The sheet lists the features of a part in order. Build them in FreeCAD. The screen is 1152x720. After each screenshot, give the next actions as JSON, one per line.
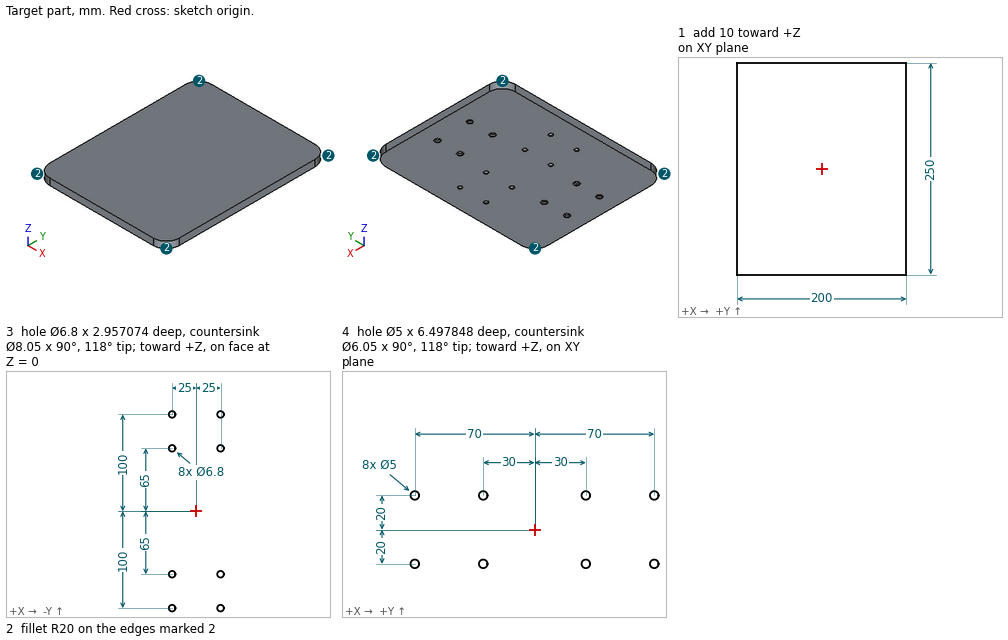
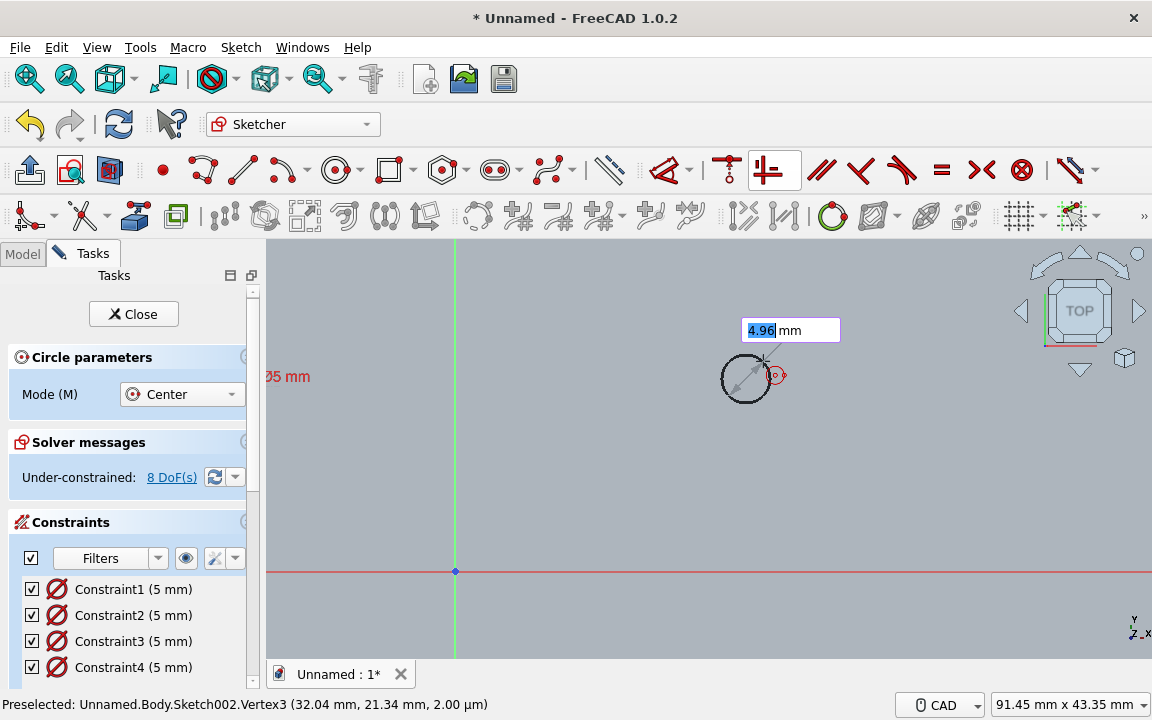
{"action": "type", "text": "5"}
{"action": "key", "text": "Return"}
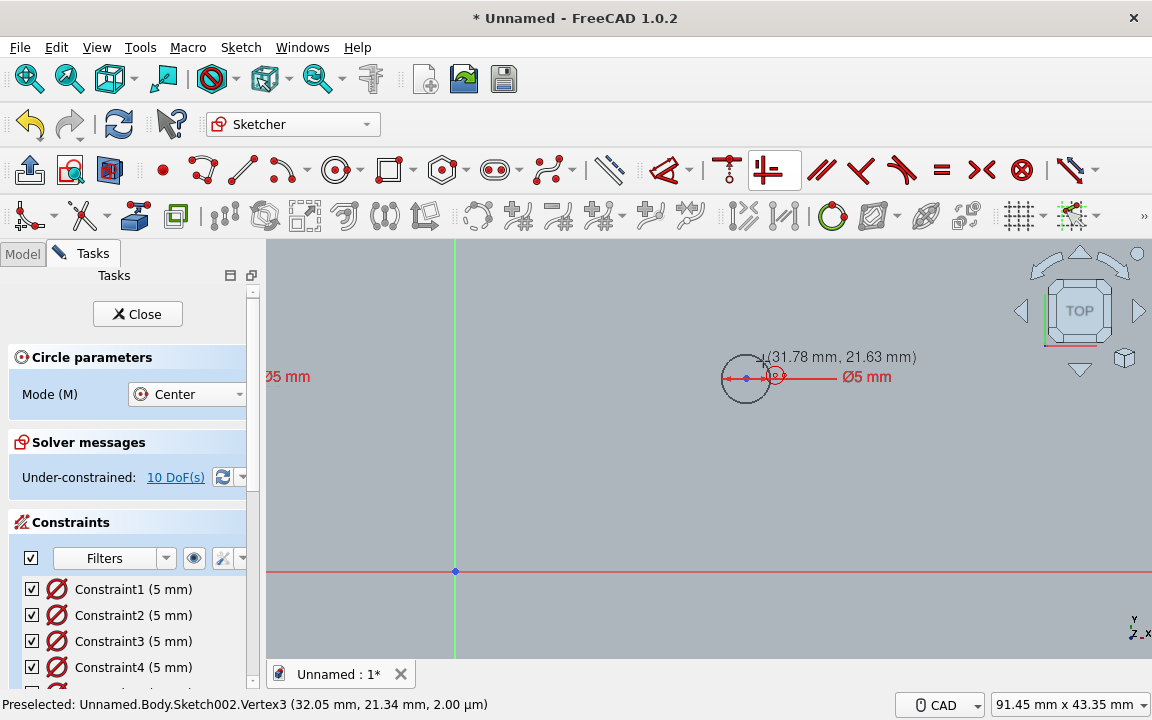
{"action": "scroll", "coordinate": [748, 378], "scroll_direction": "down", "scroll_amount": 5}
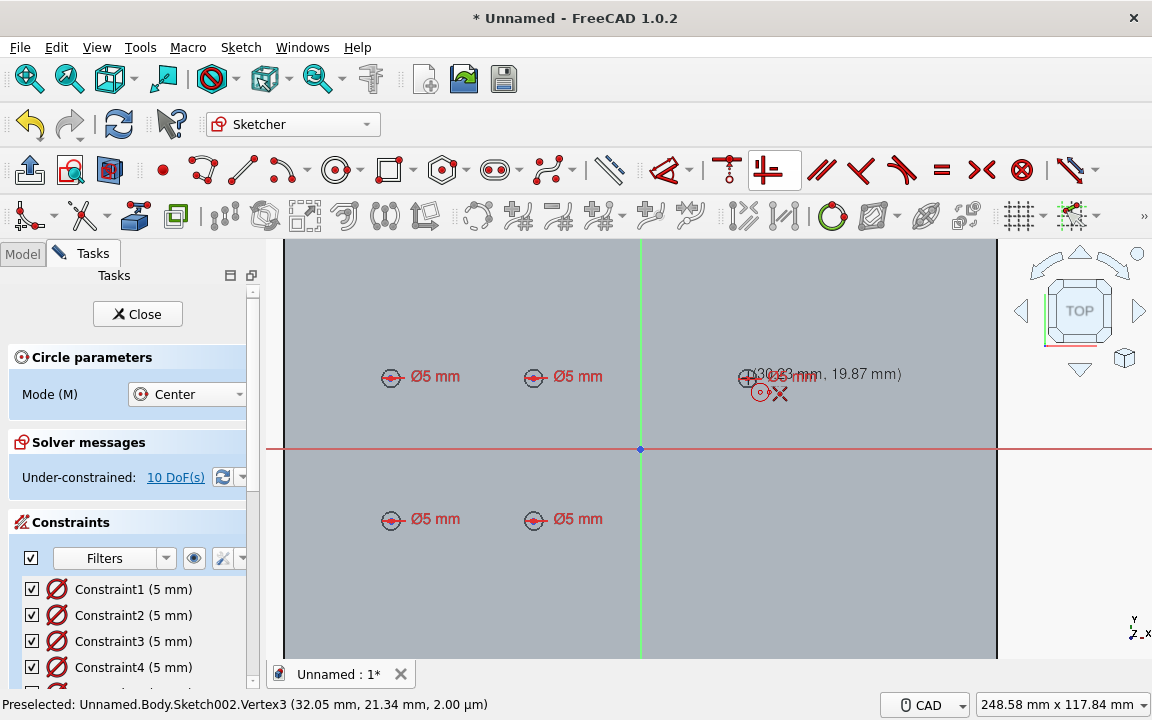
{"action": "scroll", "coordinate": [748, 521], "scroll_direction": "up", "scroll_amount": 5}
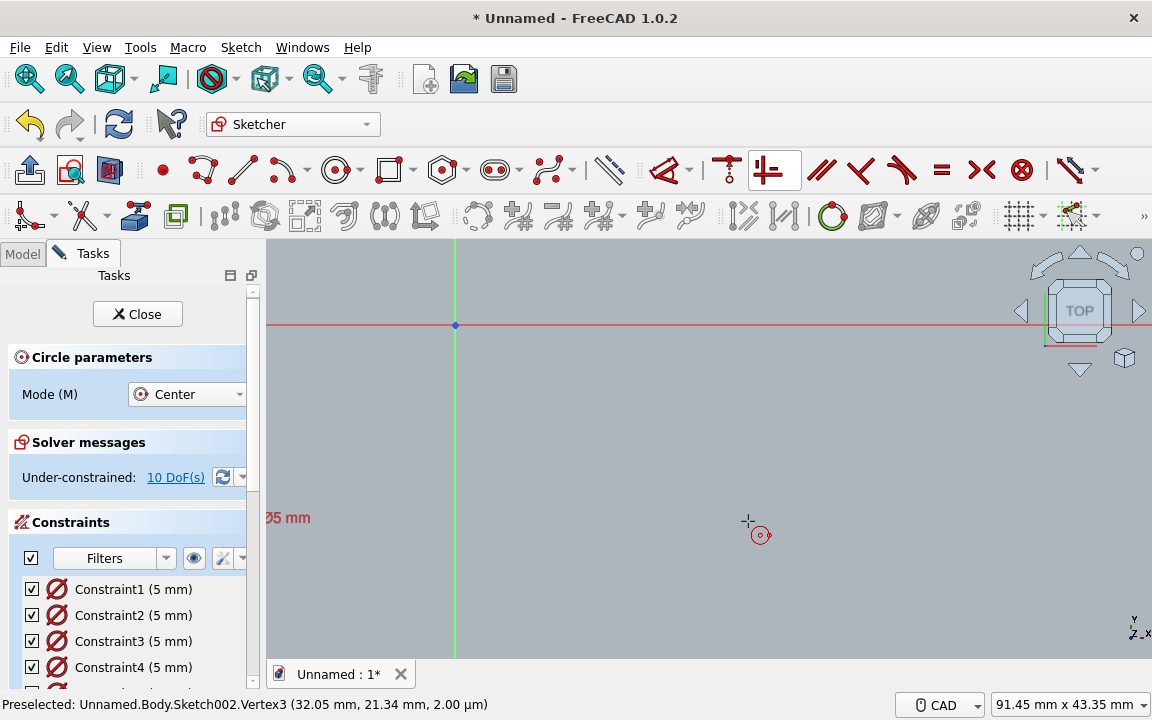
{"action": "left_click", "coordinate": [746, 519]}
{"action": "mouse_move", "coordinate": [763, 502]}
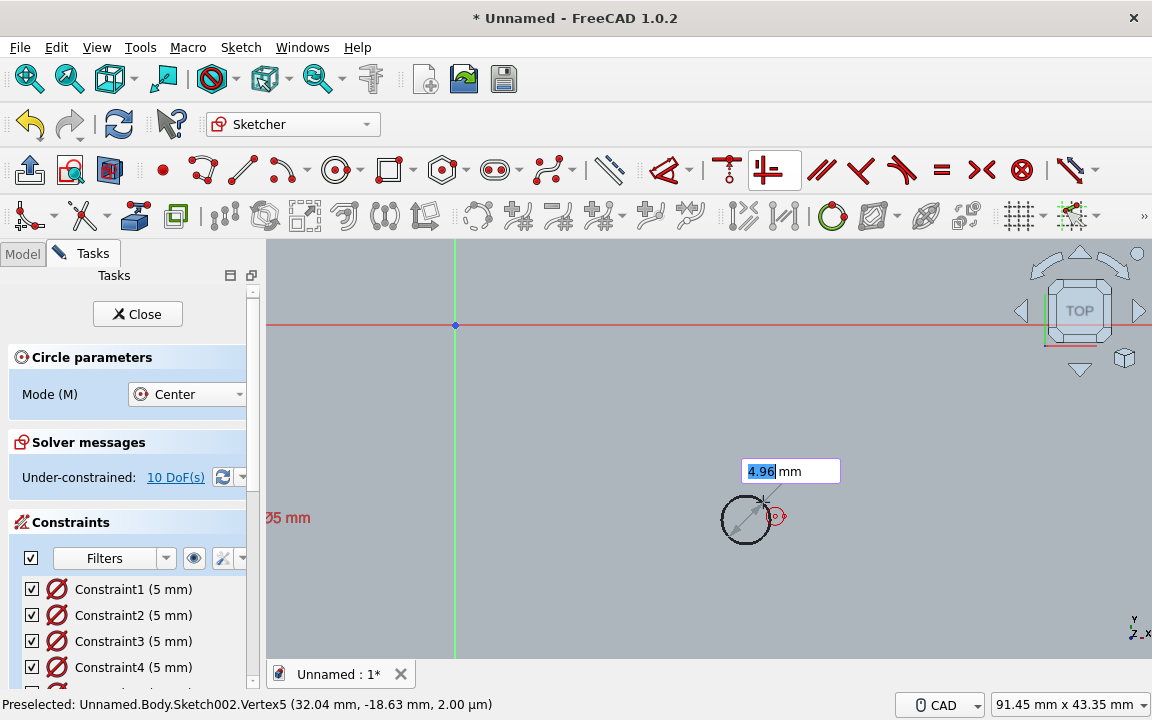
{"action": "type", "text": "5"}
{"action": "key", "text": "Return"}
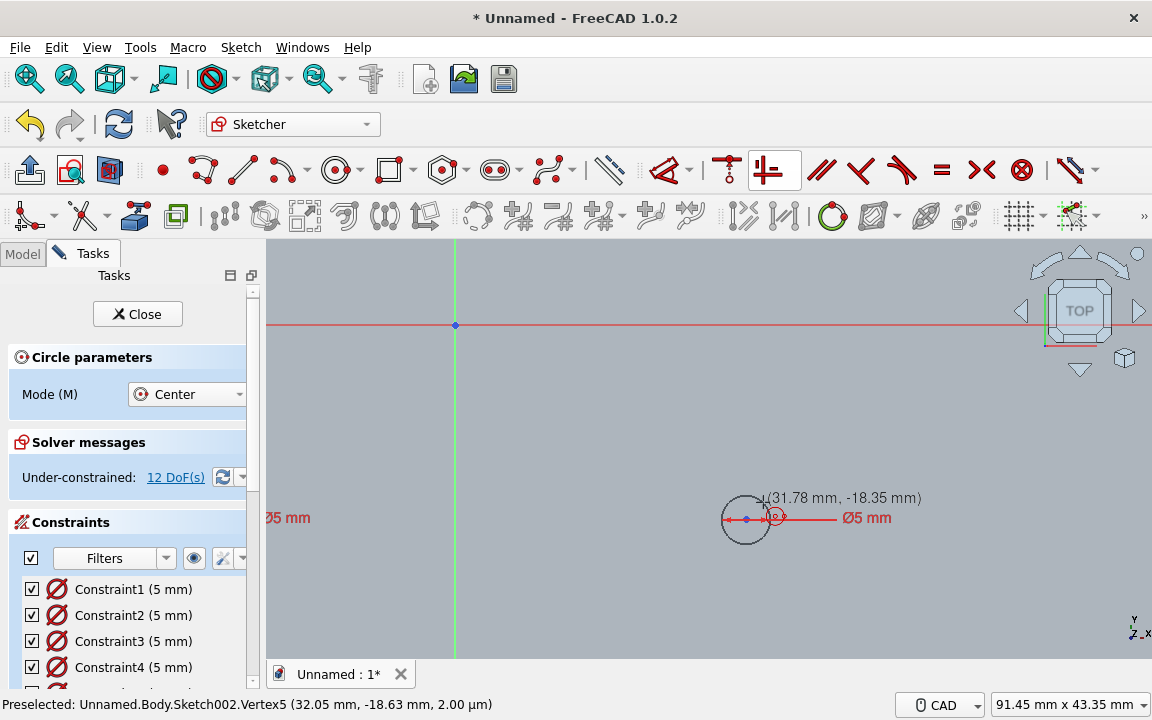
{"action": "scroll", "coordinate": [748, 521], "scroll_direction": "down", "scroll_amount": 5}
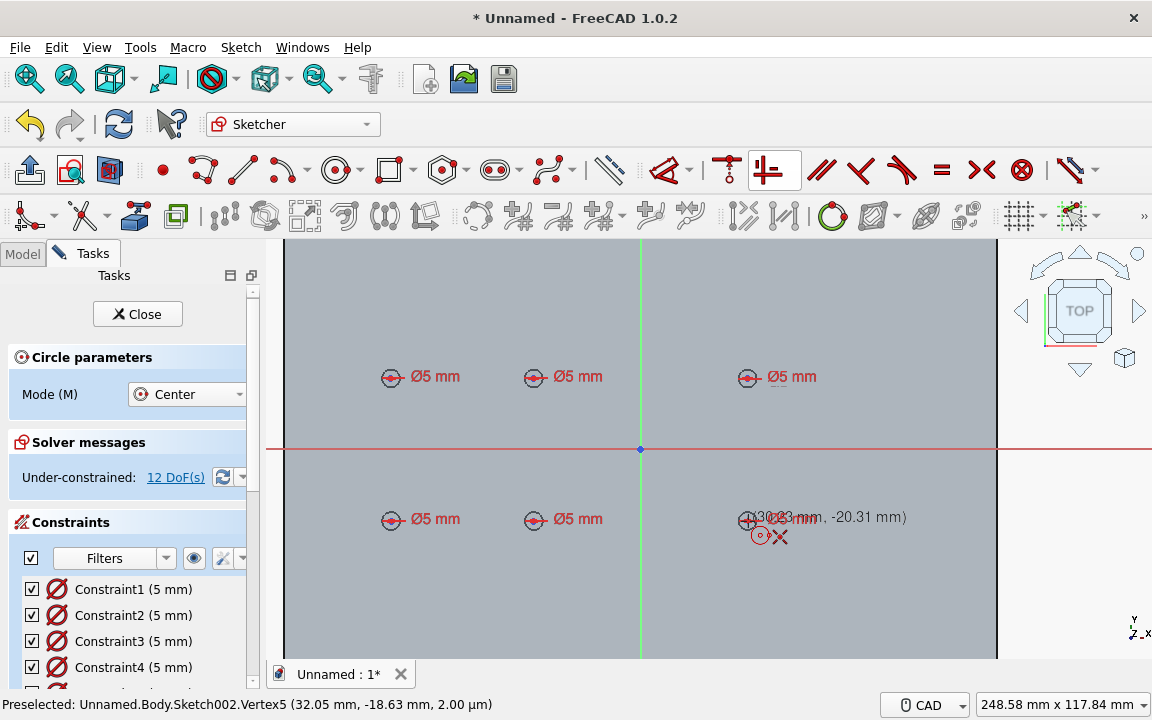
{"action": "scroll", "coordinate": [890, 378], "scroll_direction": "up", "scroll_amount": 5}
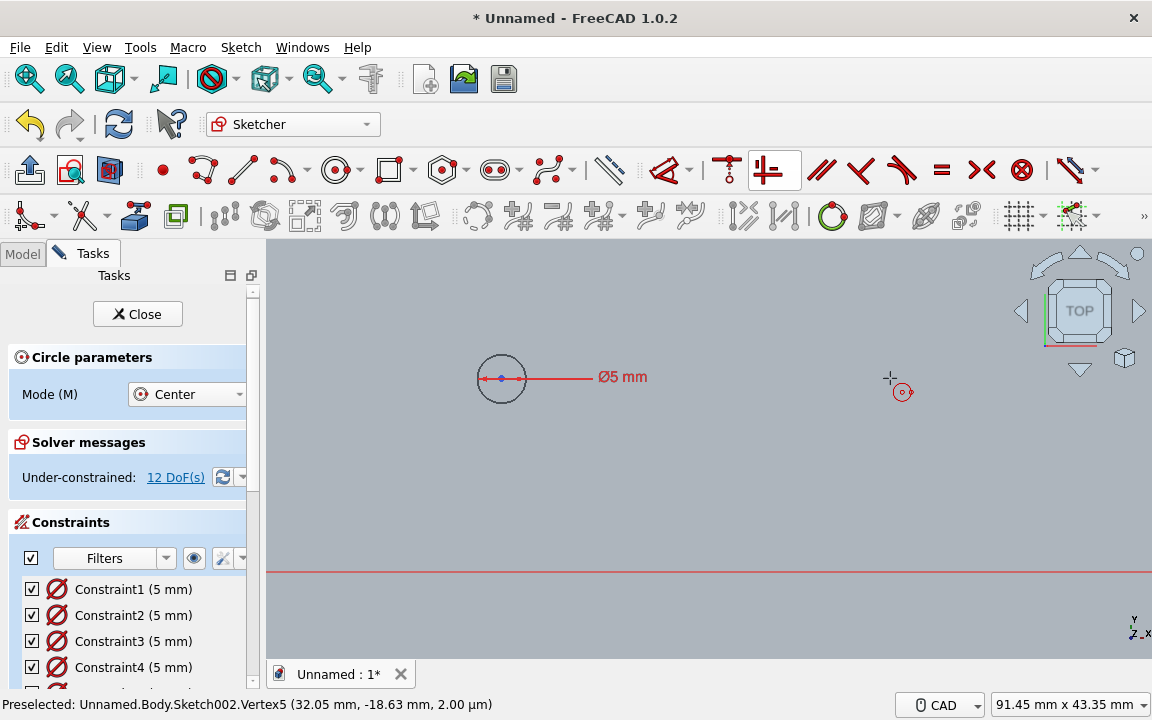
{"action": "left_click", "coordinate": [889, 378]}
{"action": "mouse_move", "coordinate": [906, 361]}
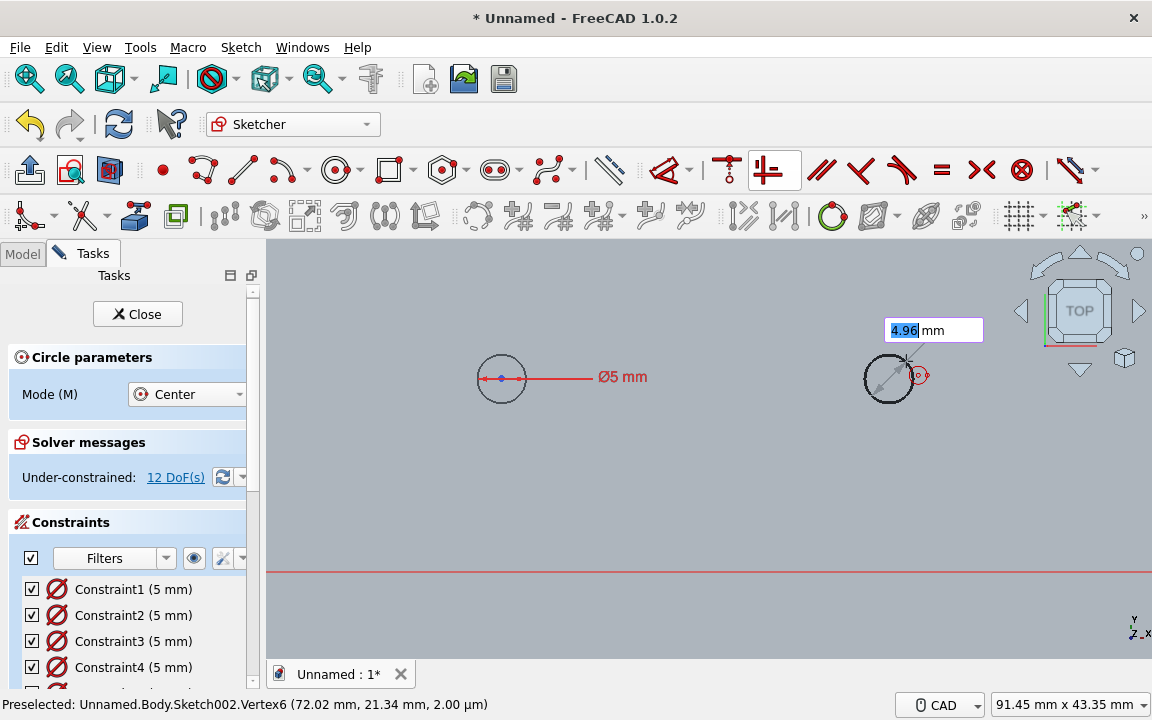
{"action": "type", "text": "5"}
{"action": "key", "text": "Return"}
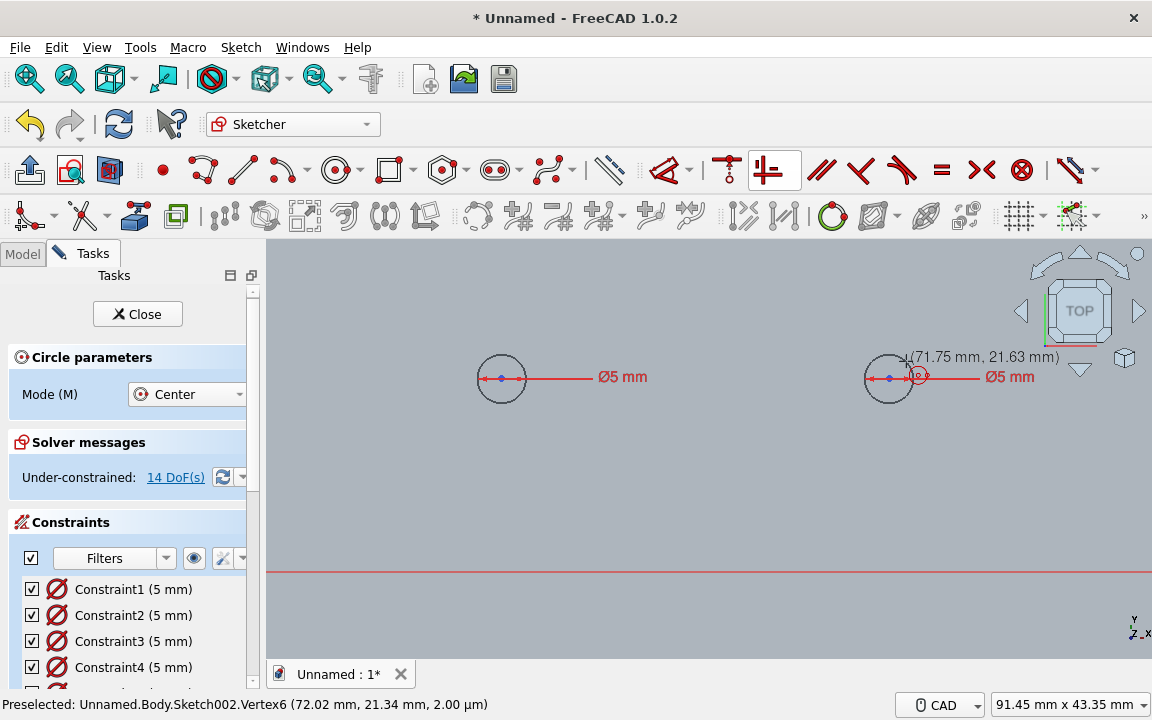
{"action": "scroll", "coordinate": [891, 378], "scroll_direction": "down", "scroll_amount": 5}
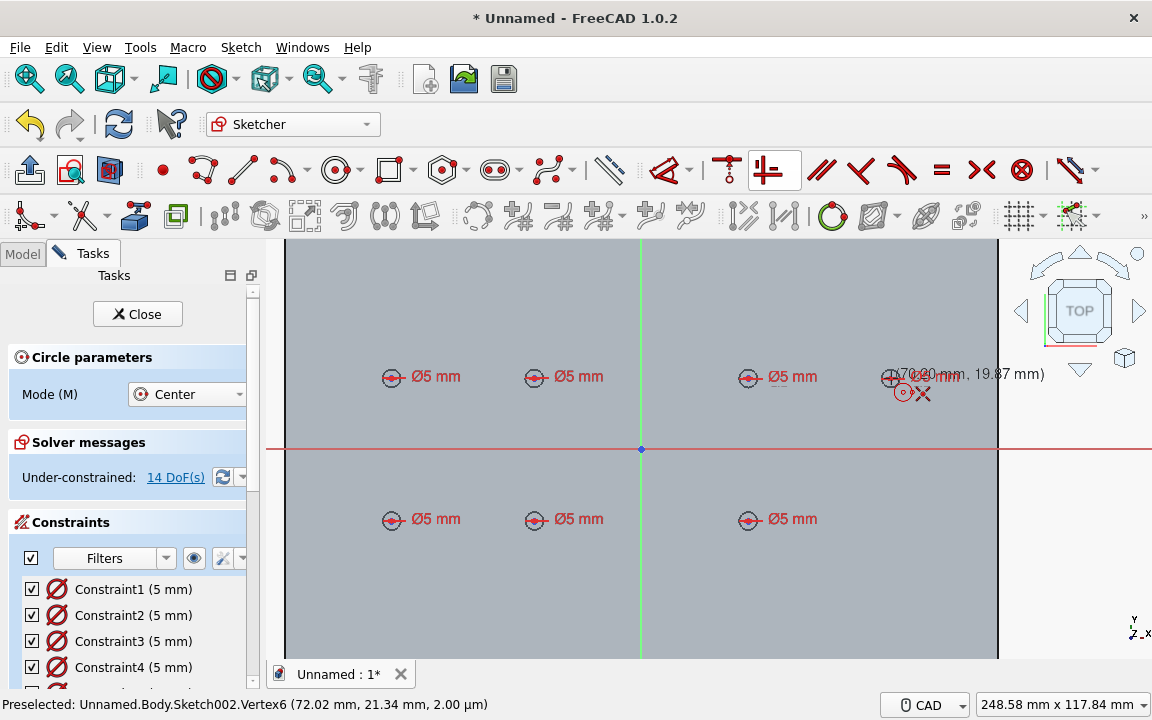
{"action": "scroll", "coordinate": [891, 521], "scroll_direction": "up", "scroll_amount": 5}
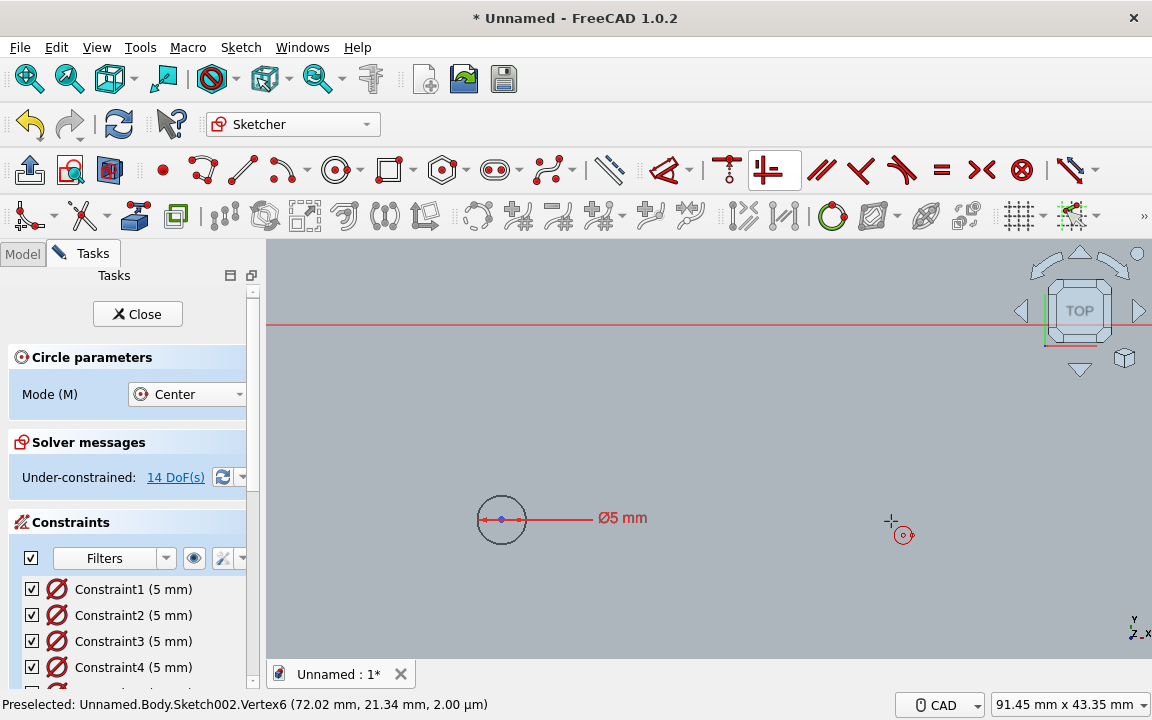
{"action": "left_click", "coordinate": [889, 519]}
{"action": "mouse_move", "coordinate": [906, 502]}